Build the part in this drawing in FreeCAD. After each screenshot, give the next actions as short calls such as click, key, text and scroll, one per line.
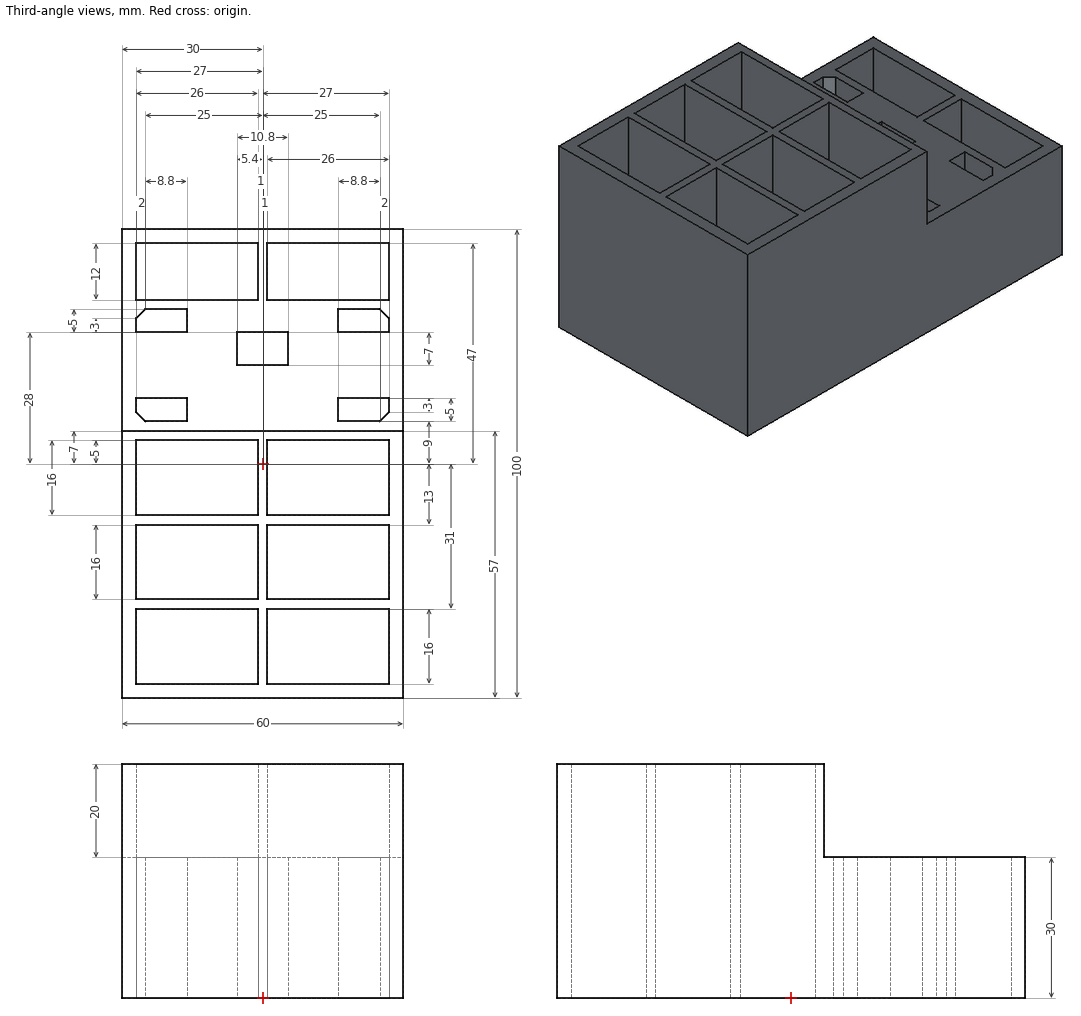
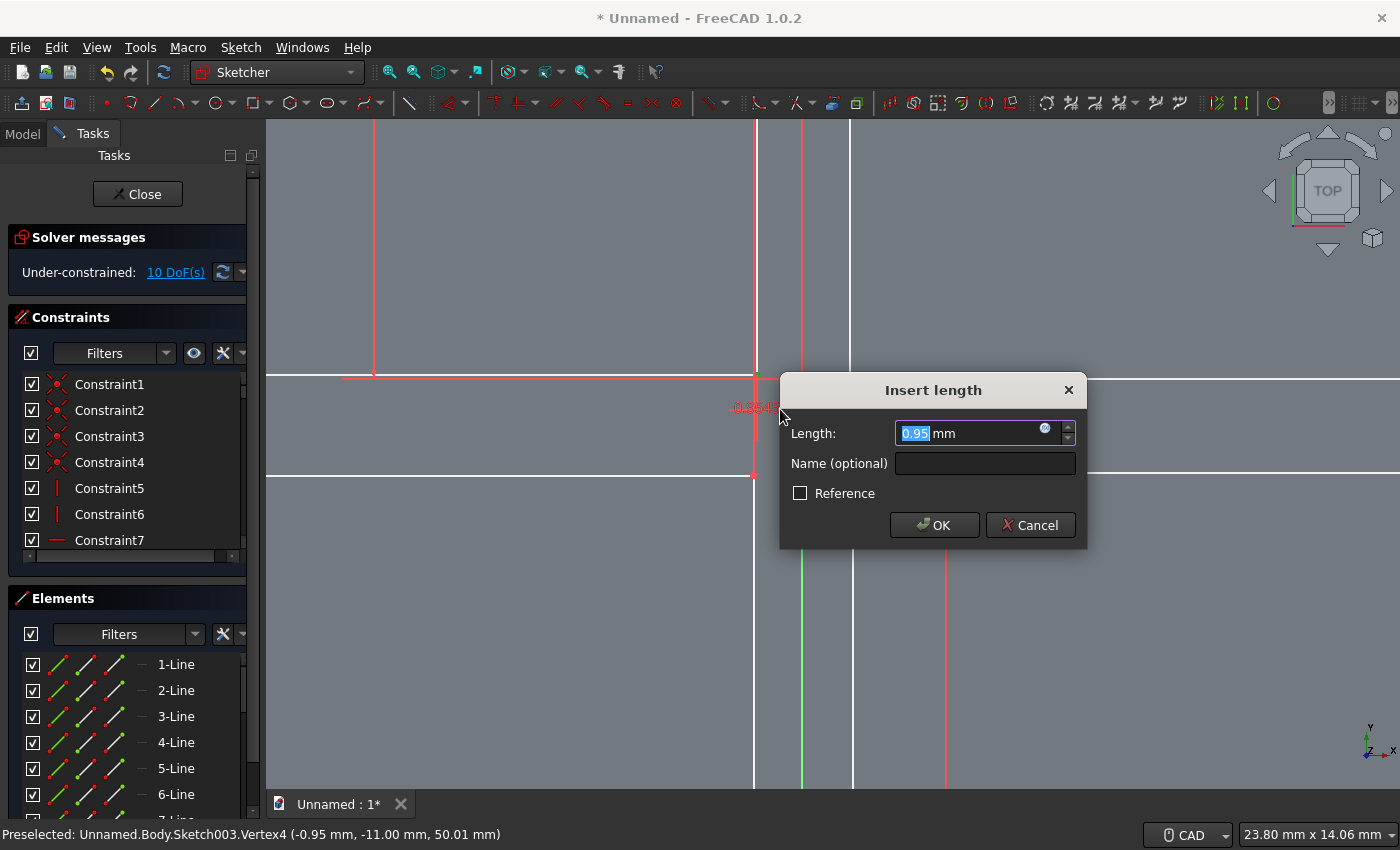
text(1)
key(Return)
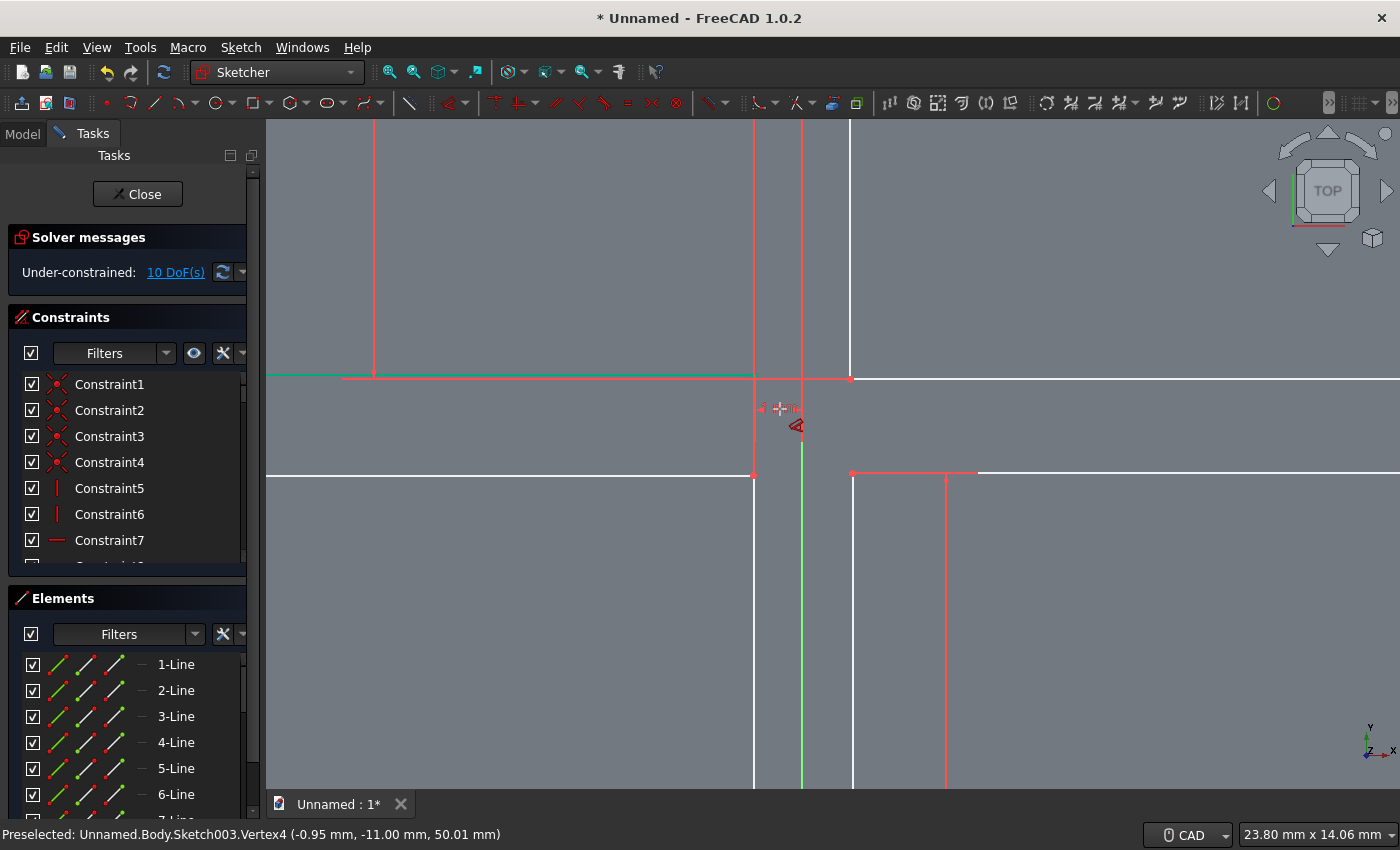
scroll(757, 375, down, 9)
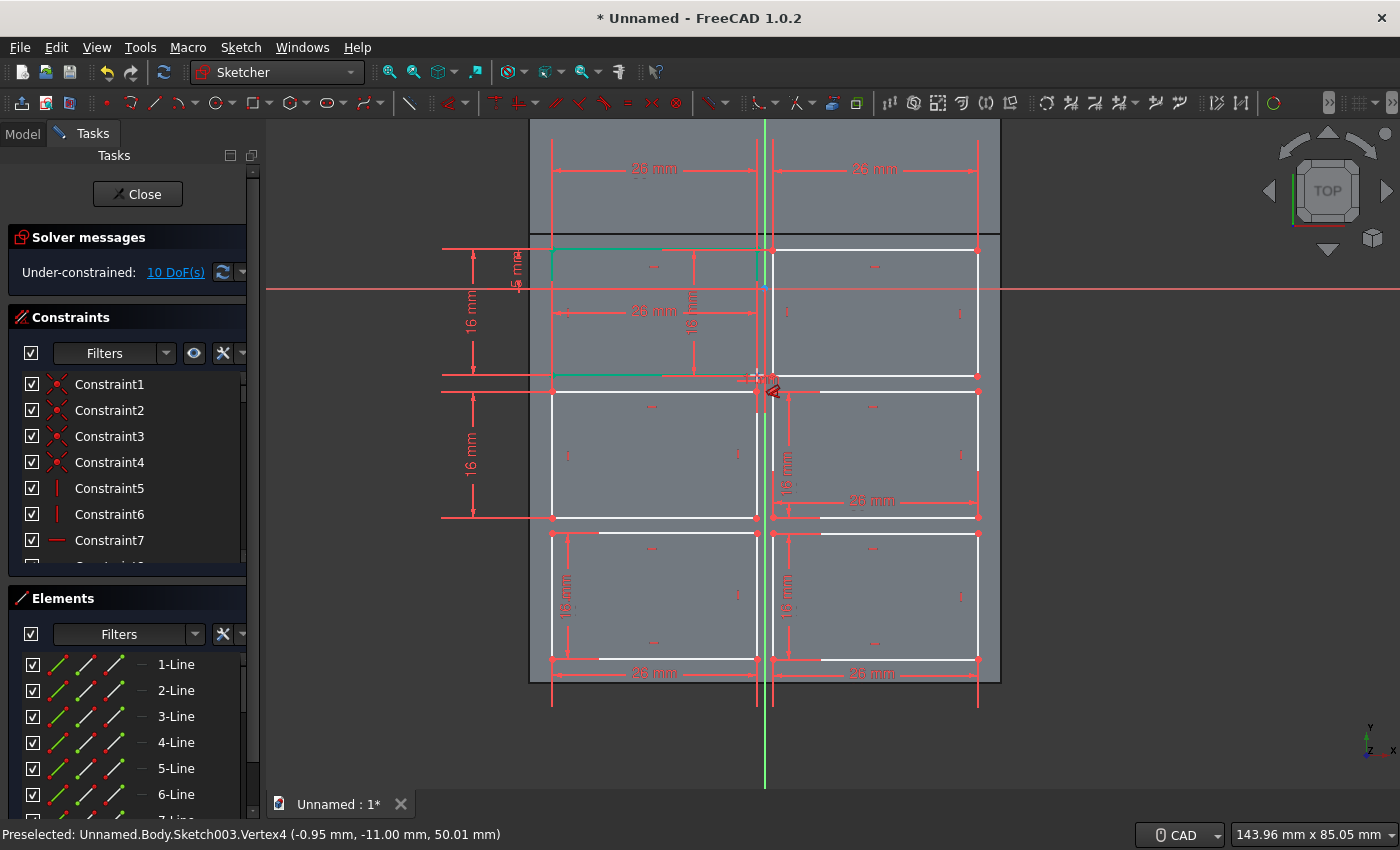
scroll(773, 250, up, 9)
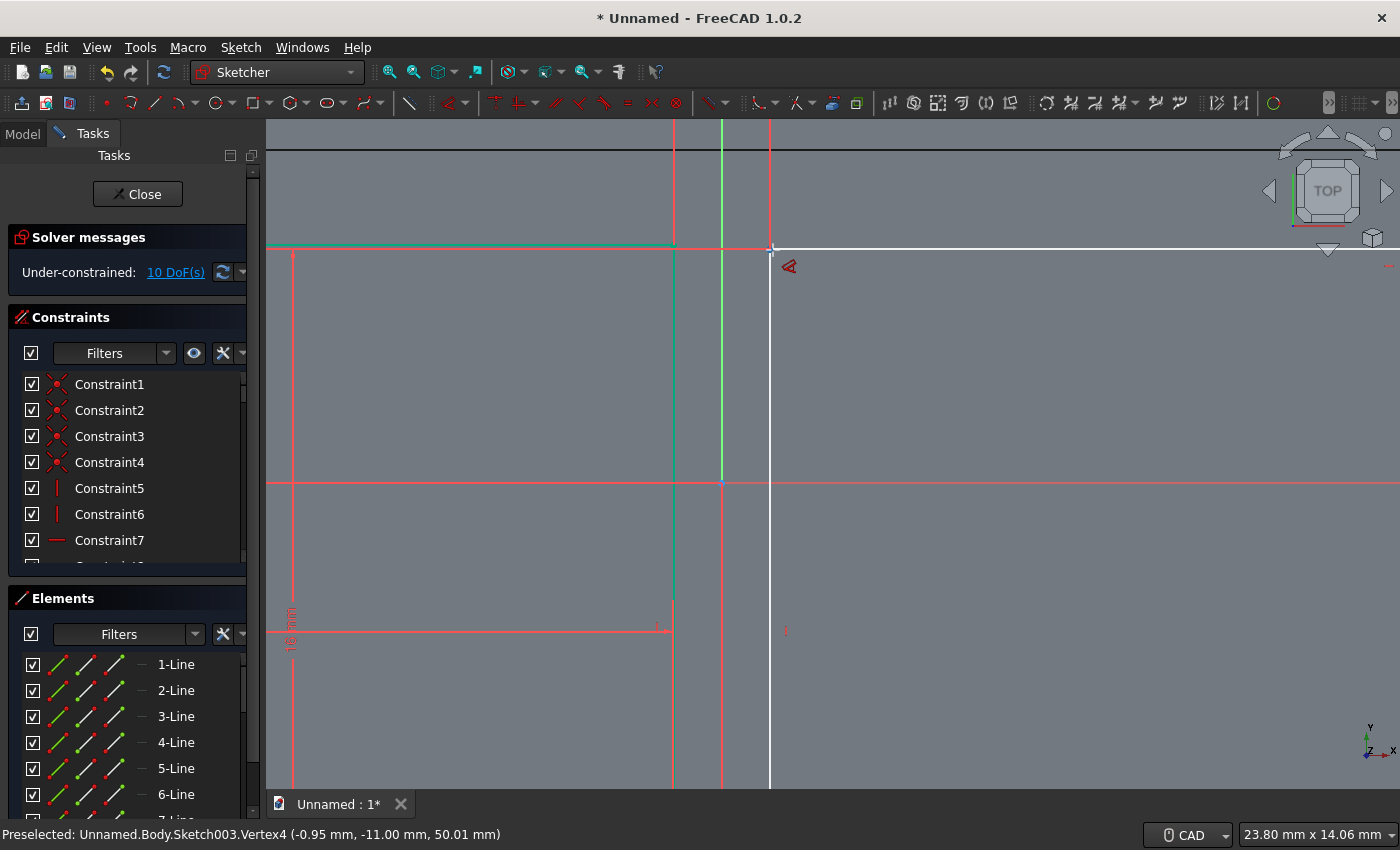
click(770, 249)
click(746, 215)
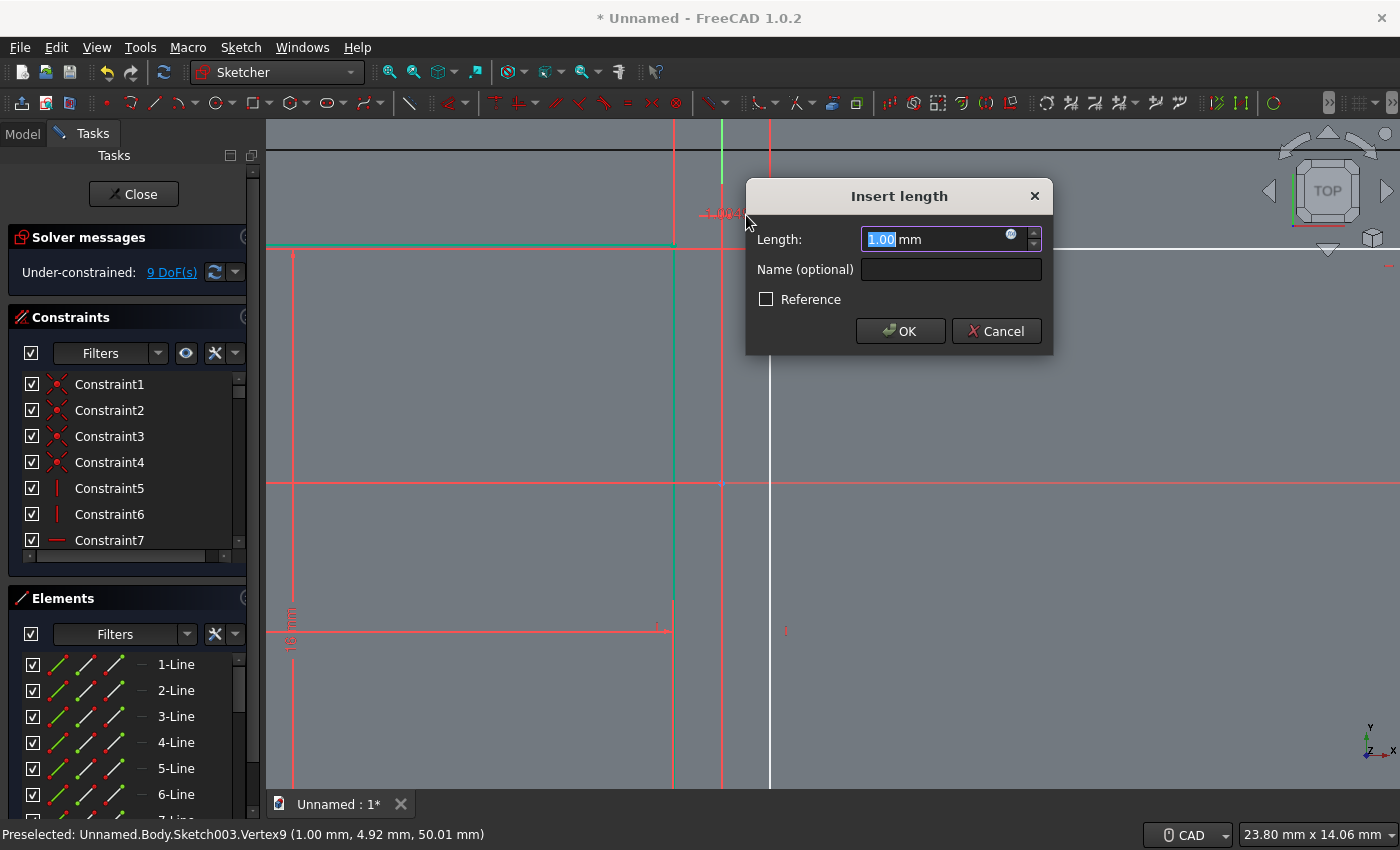
text(1)
key(Return)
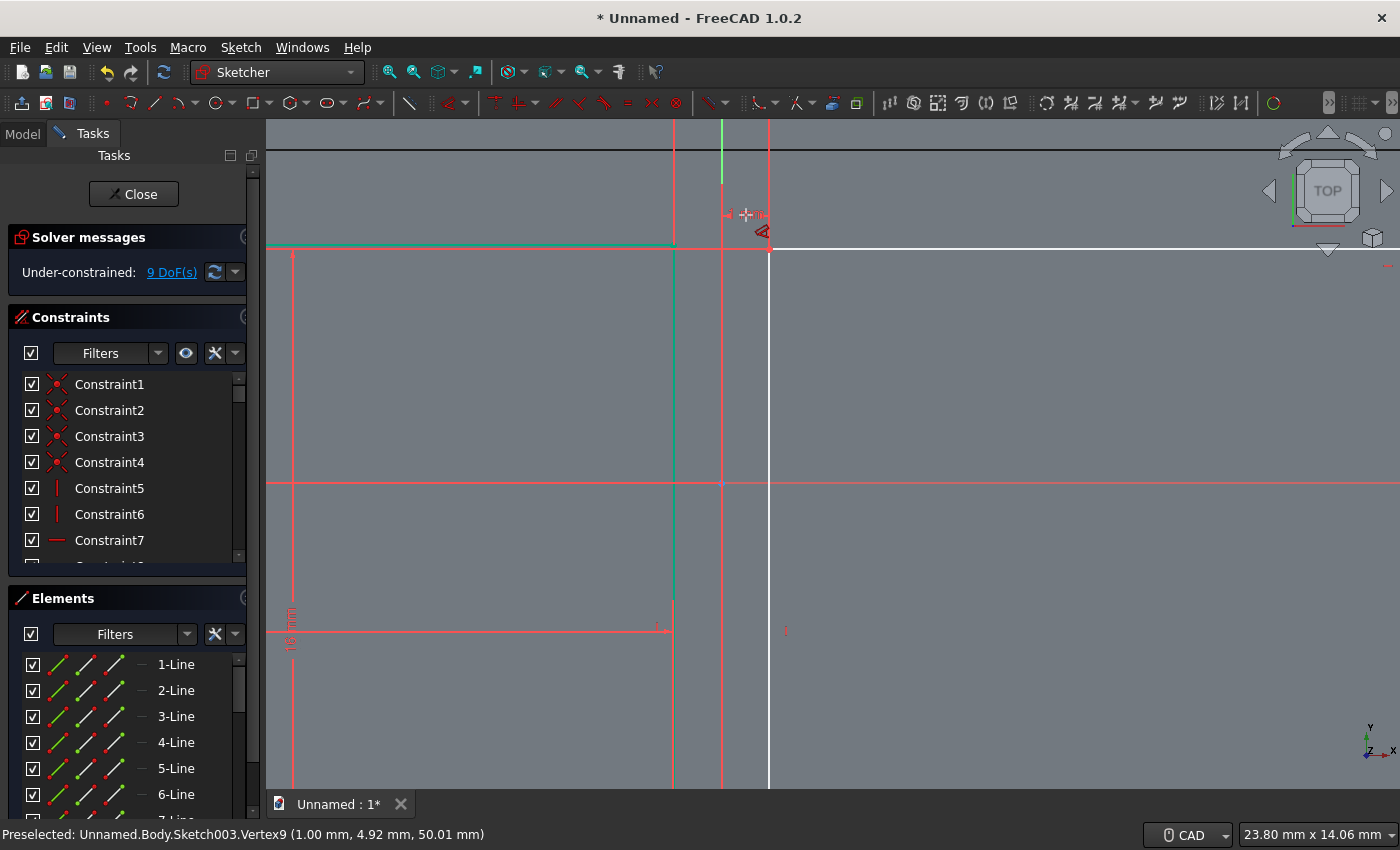
scroll(773, 250, down, 9)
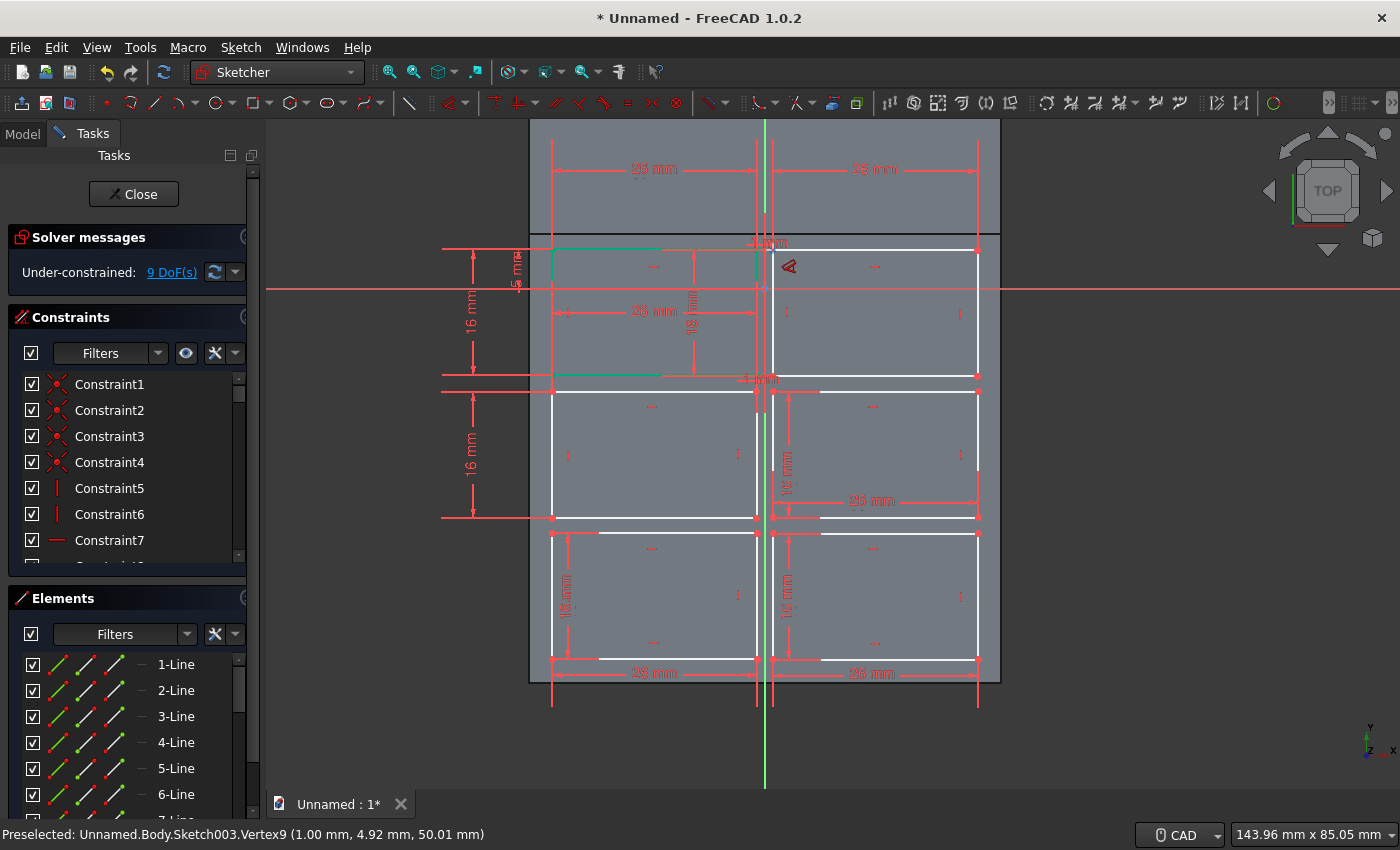
click(773, 250)
click(807, 269)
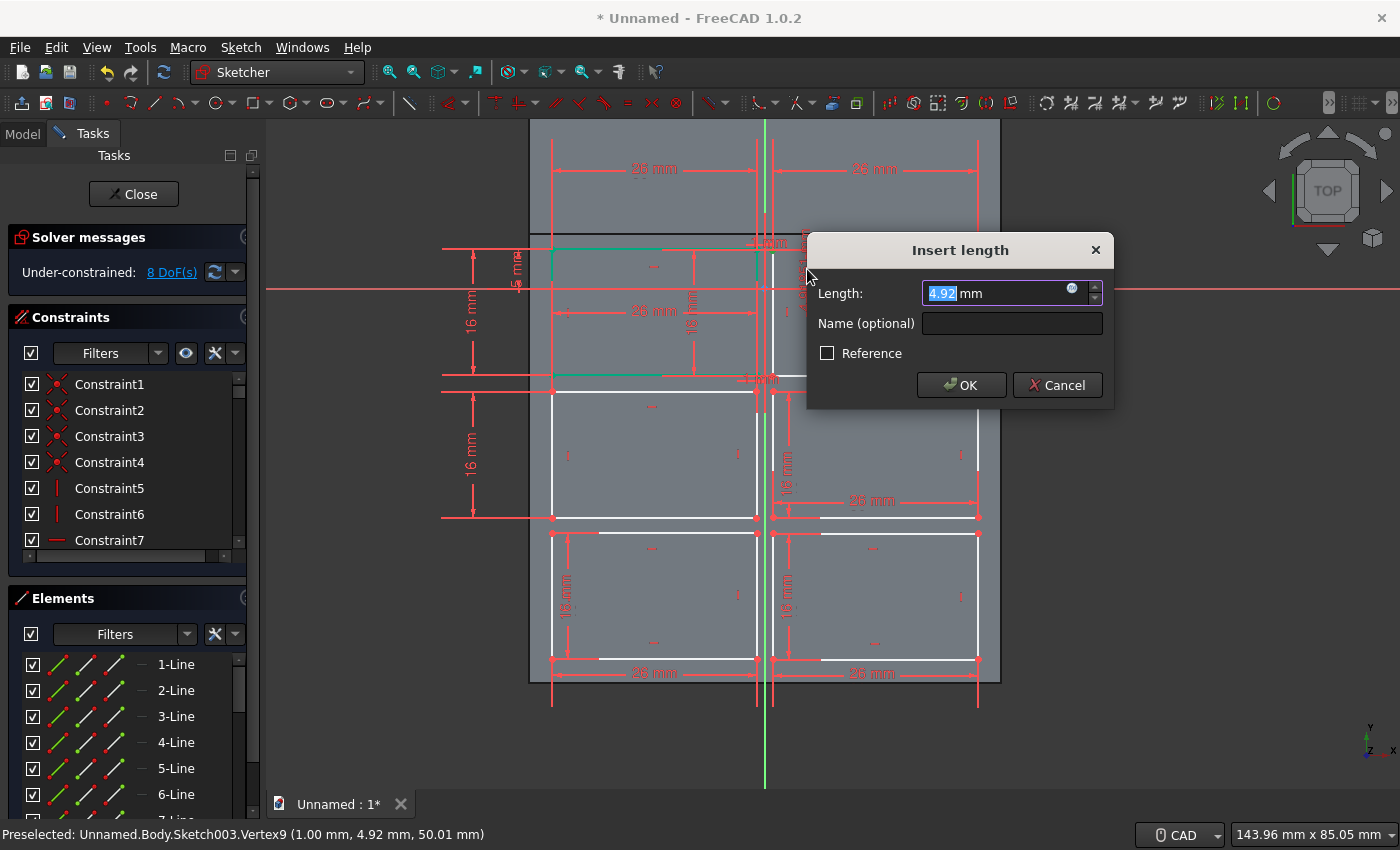
text(5)
key(Return)